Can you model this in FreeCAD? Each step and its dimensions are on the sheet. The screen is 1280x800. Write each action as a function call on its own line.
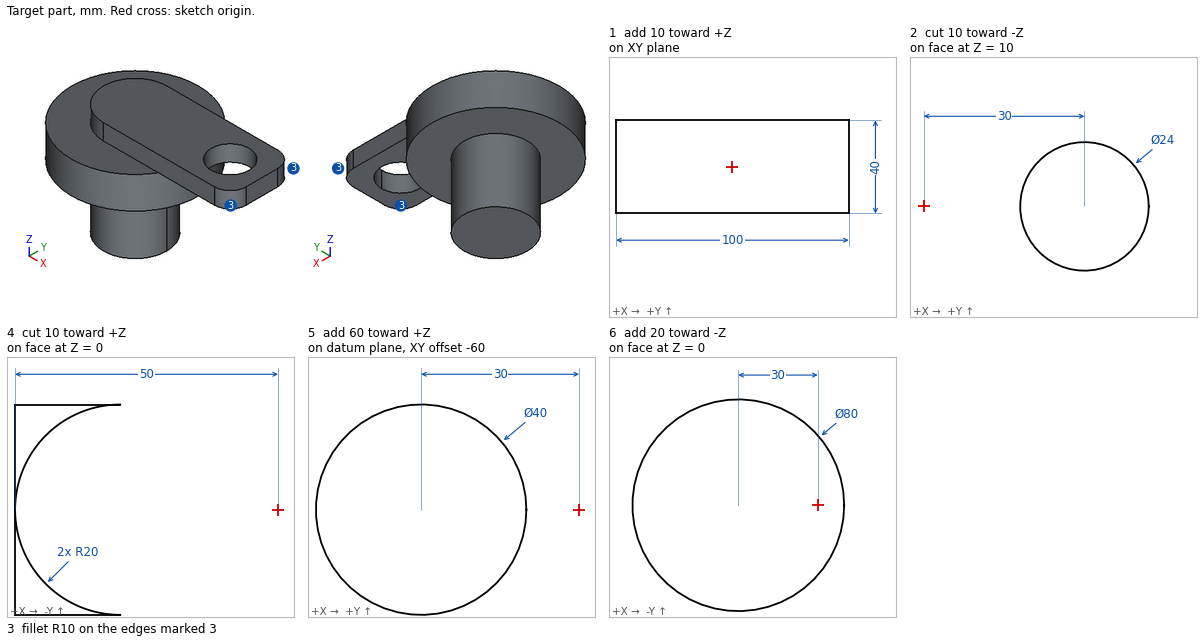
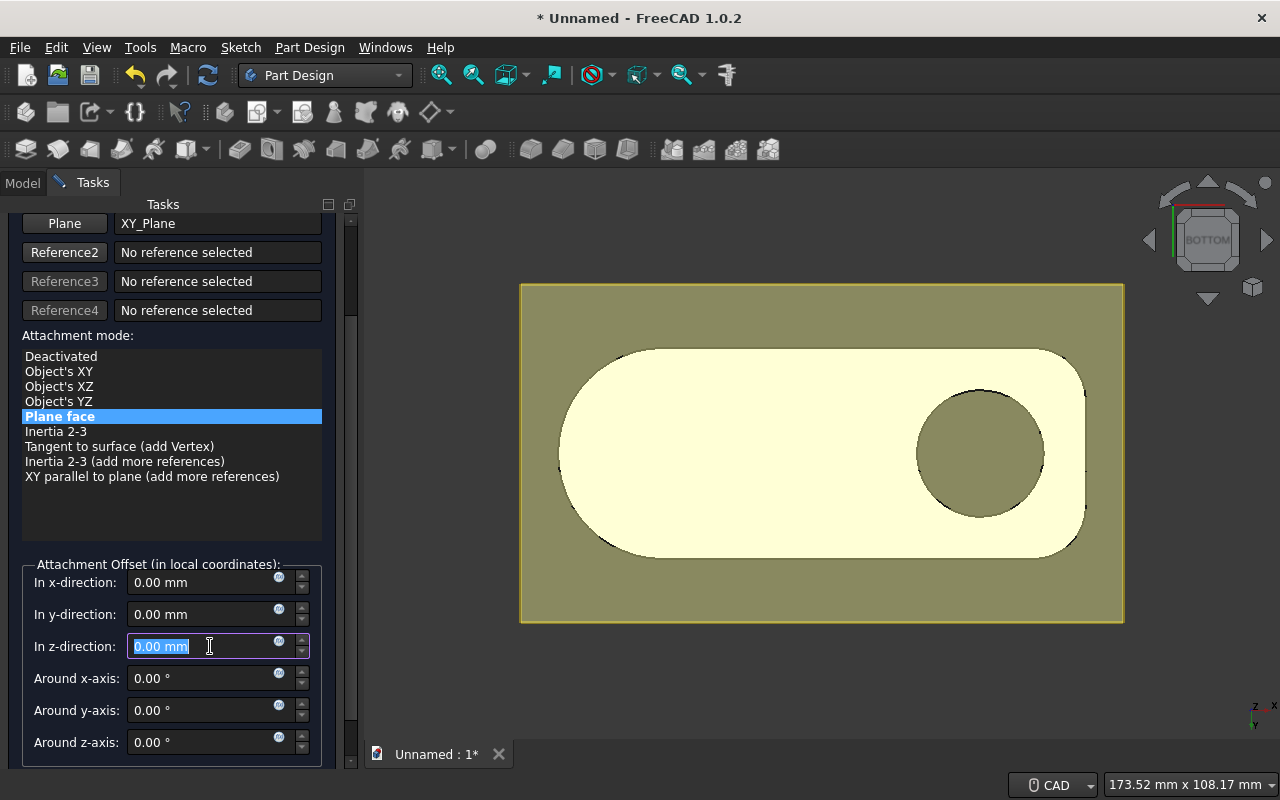
text(-60)
key(Tab)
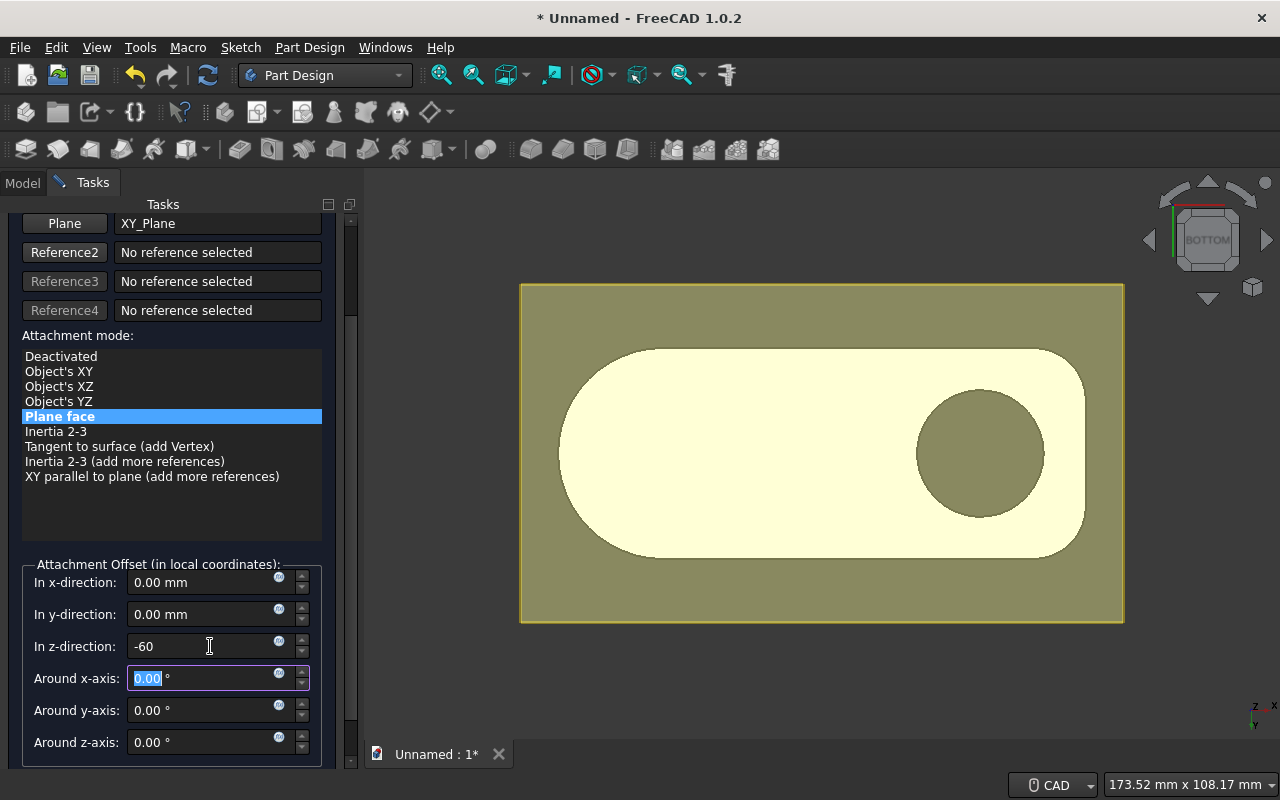
scroll(351, 491, up, 3)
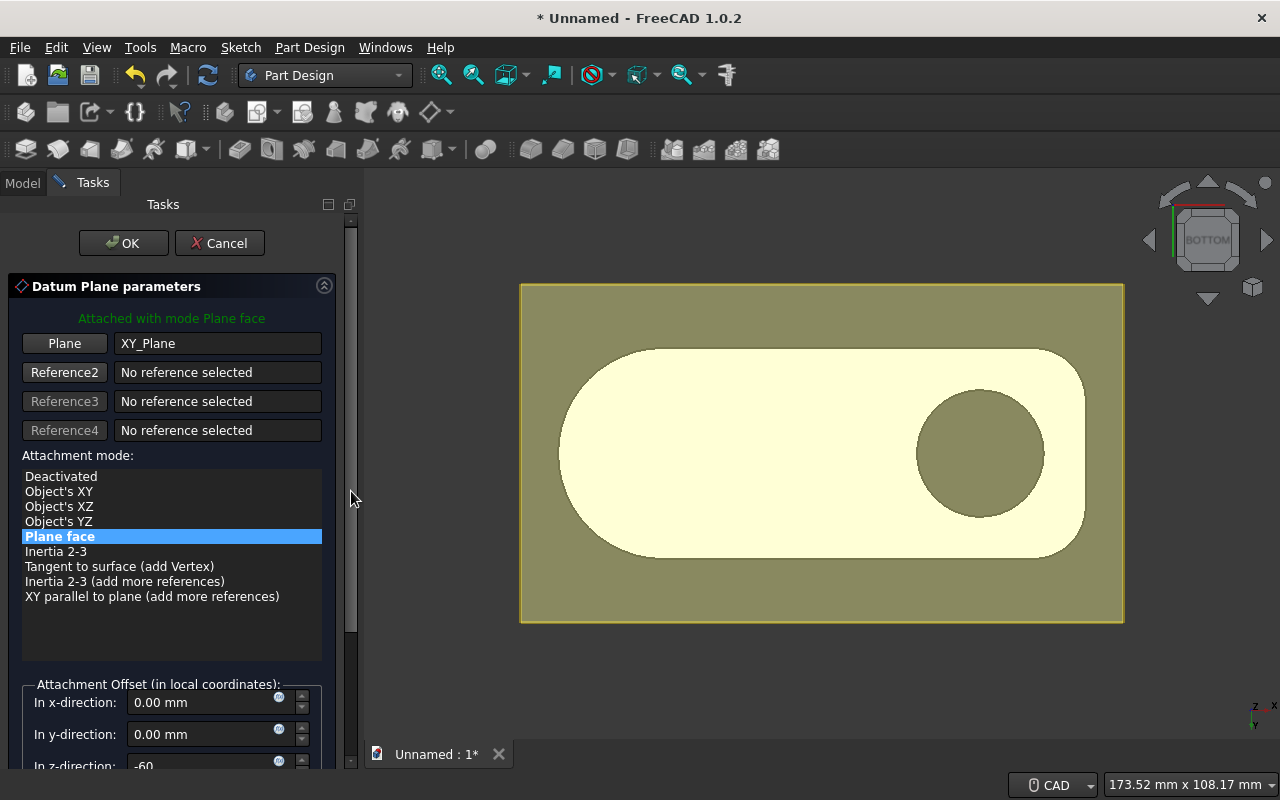
click(124, 243)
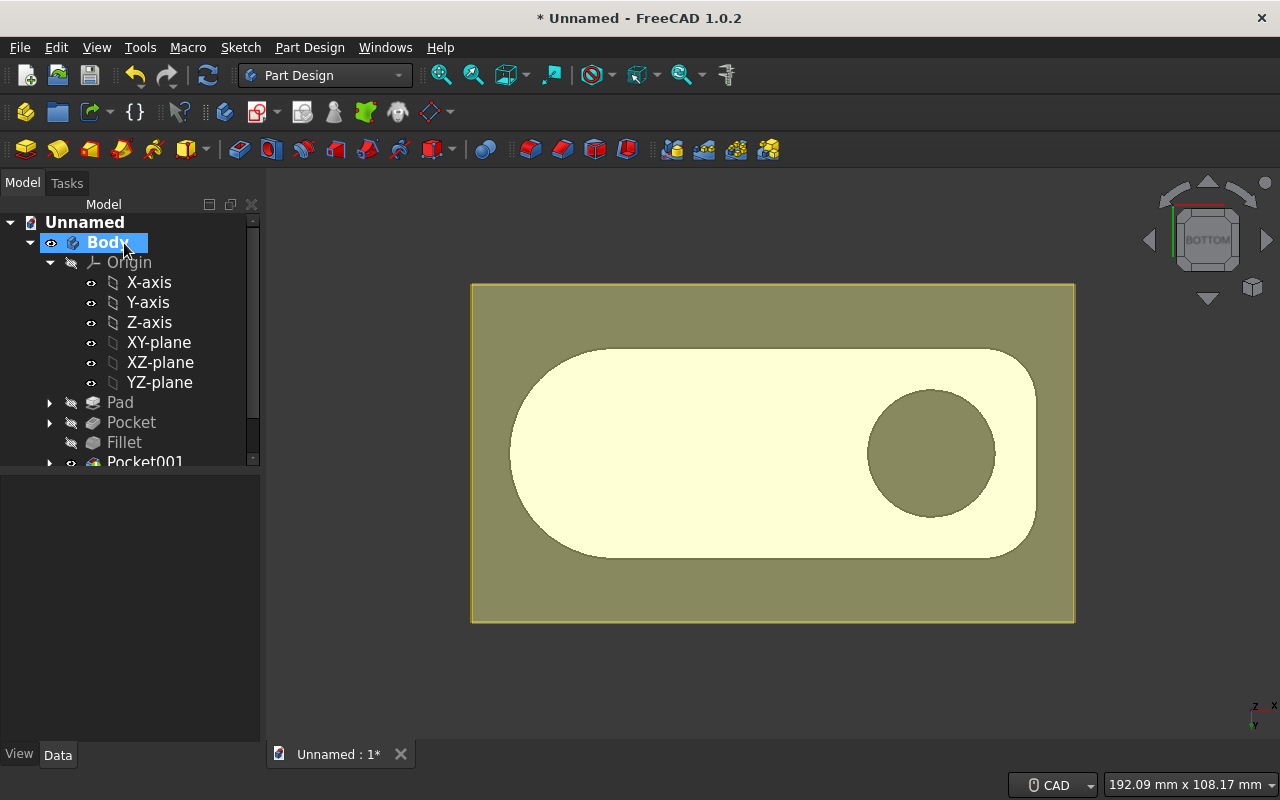
scroll(100, 338, down, 3)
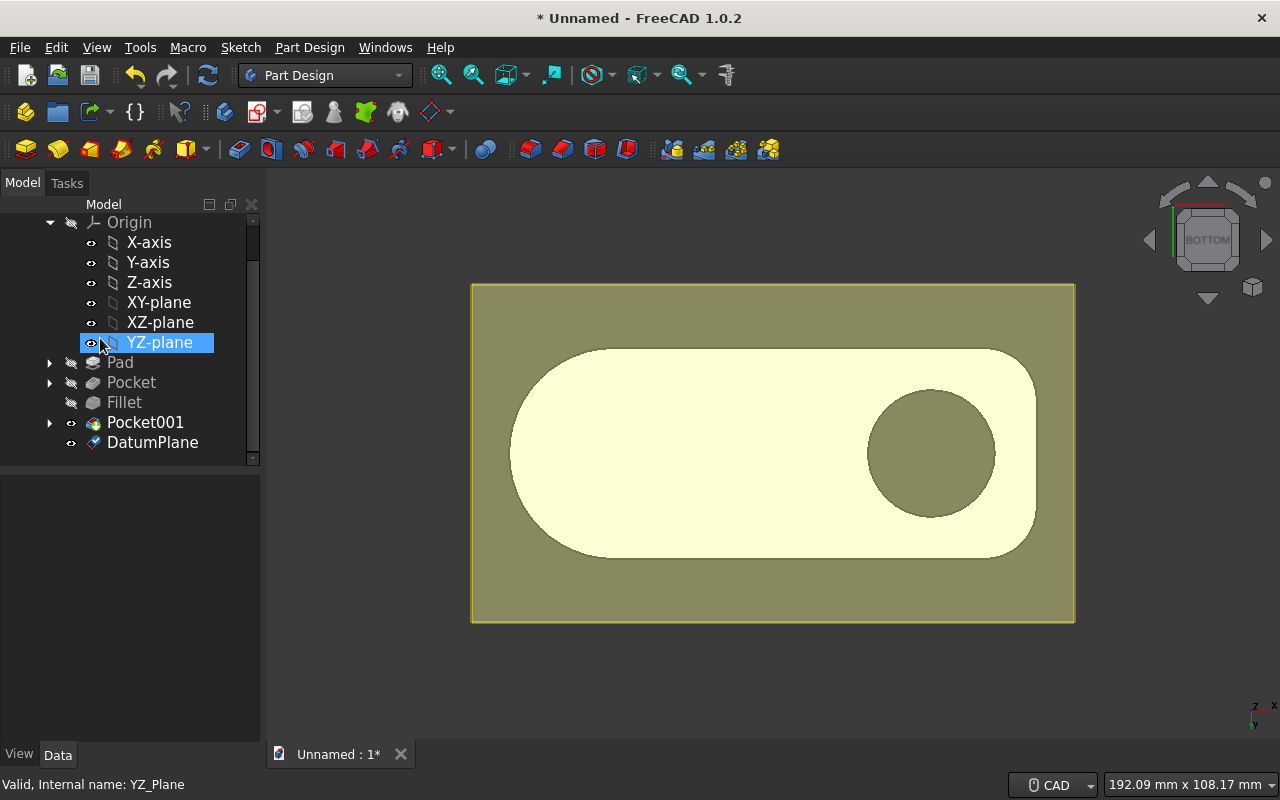
click(116, 443)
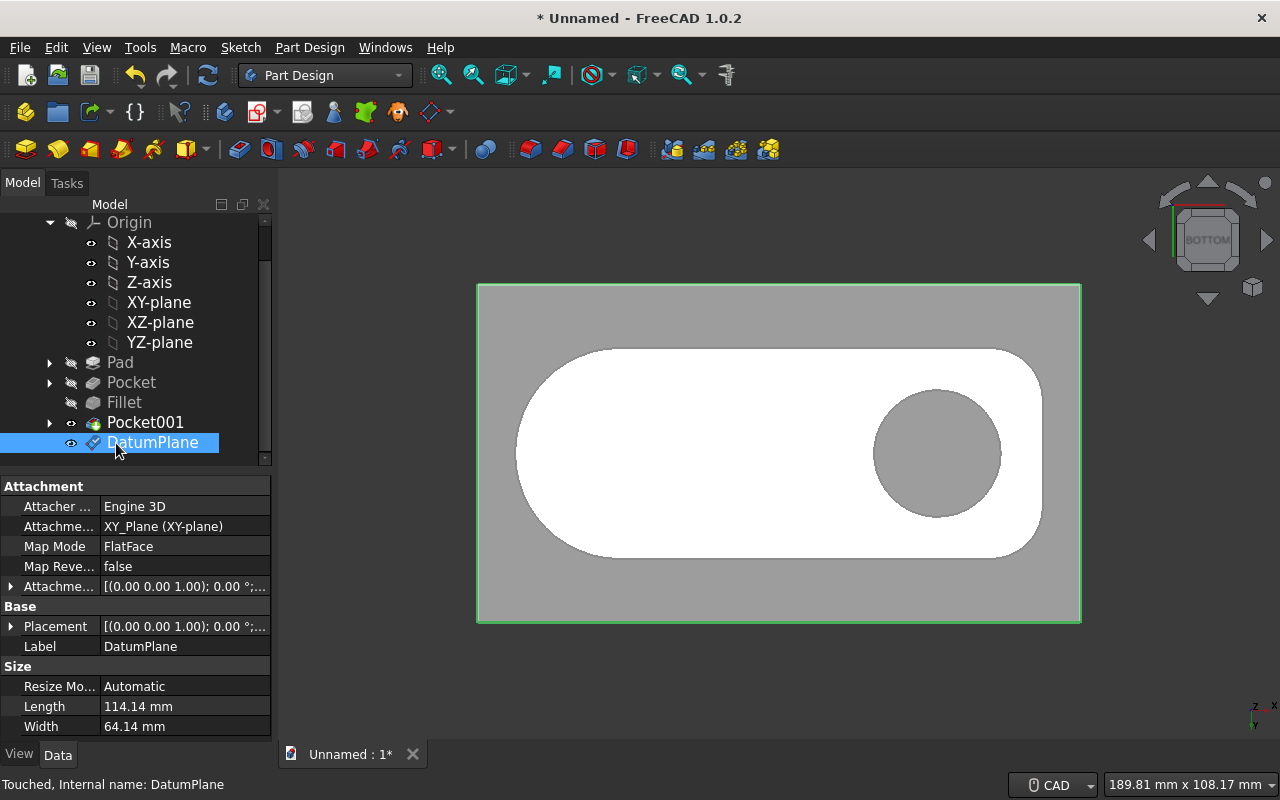
click(258, 112)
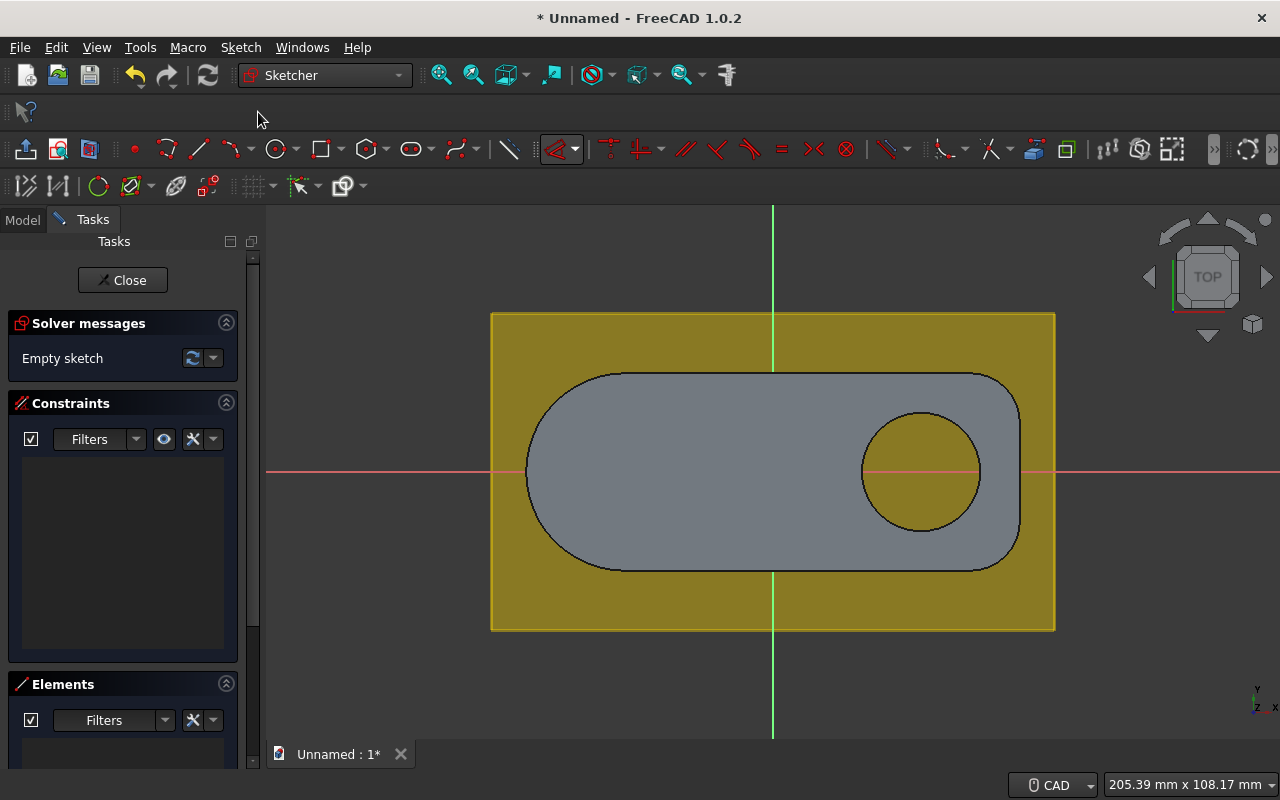
key(q)
key(s)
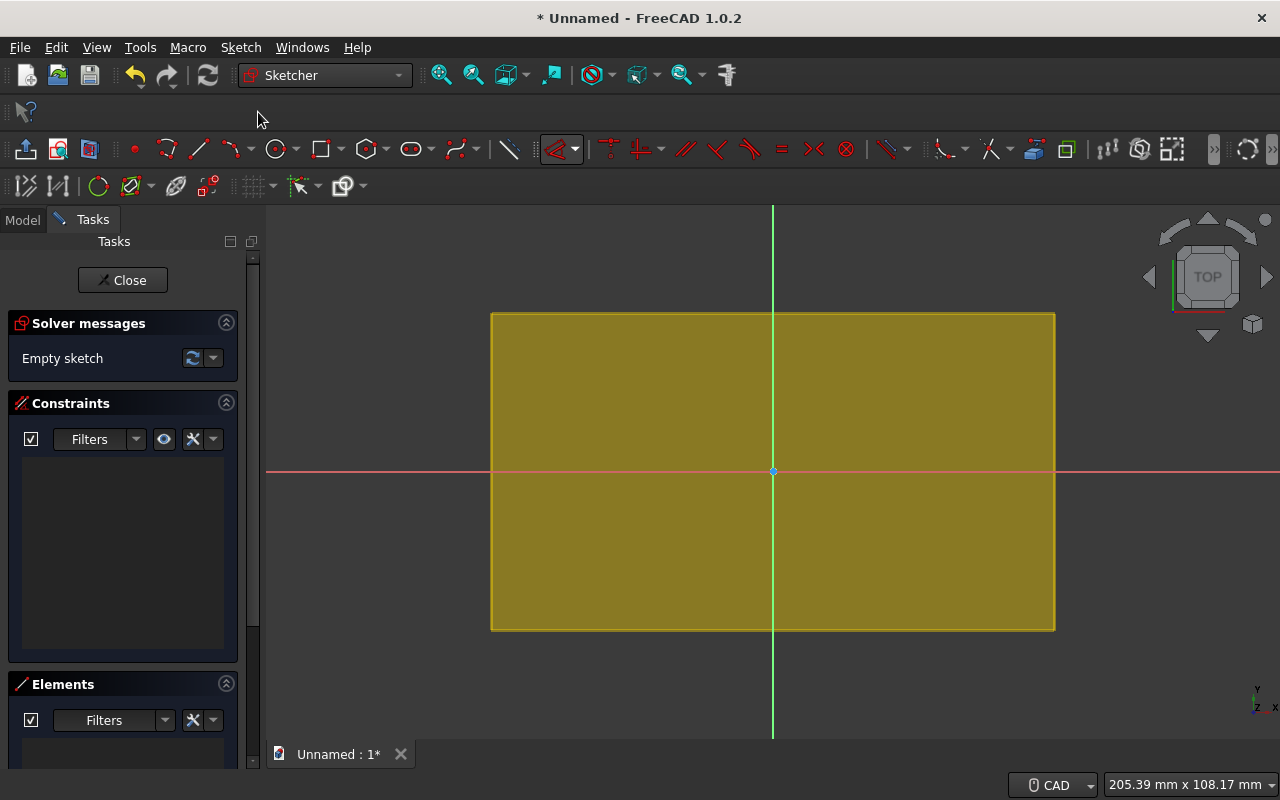
scroll(583, 472, up, 3)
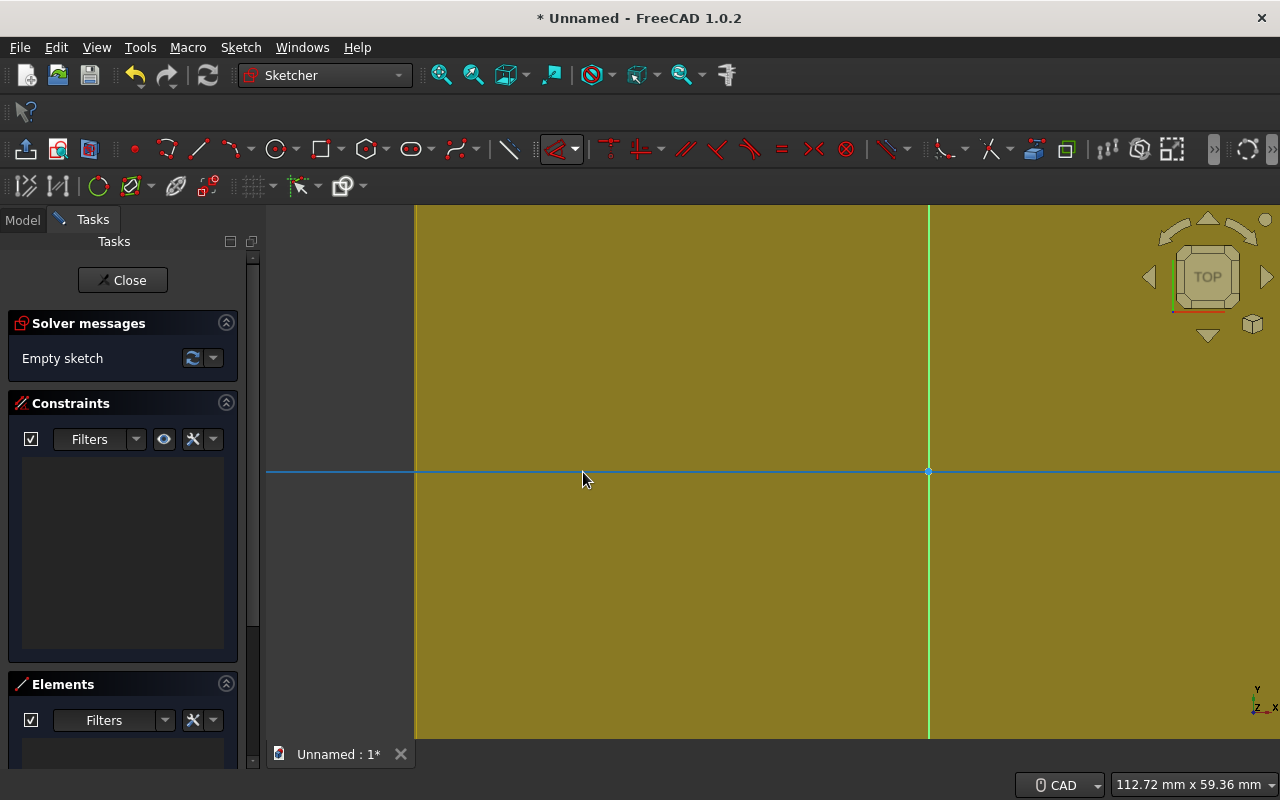
key(g)
key(c)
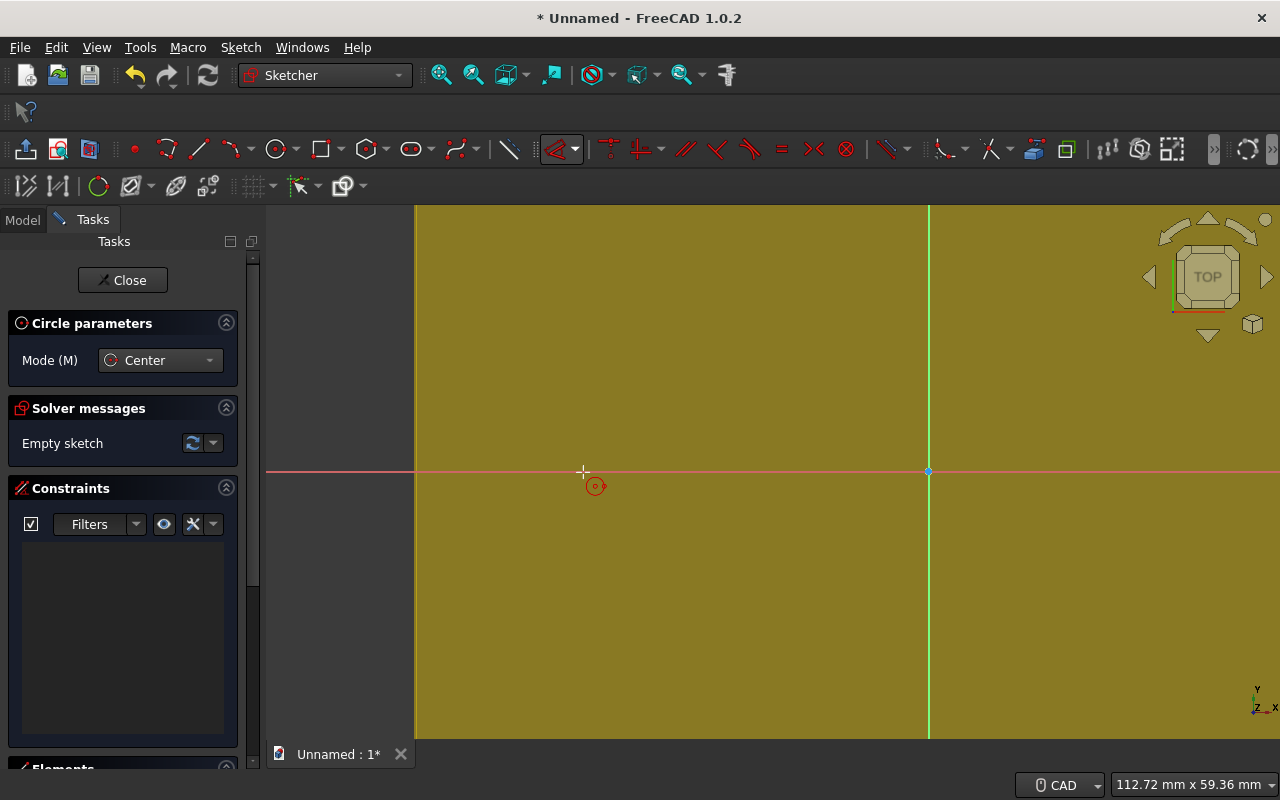
click(659, 472)
move(786, 344)